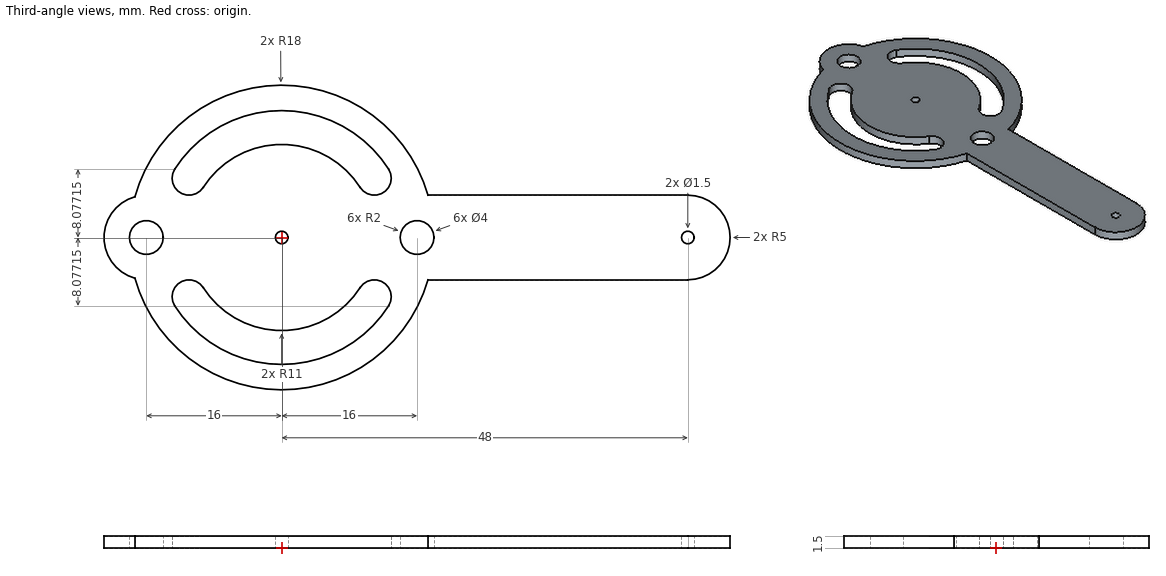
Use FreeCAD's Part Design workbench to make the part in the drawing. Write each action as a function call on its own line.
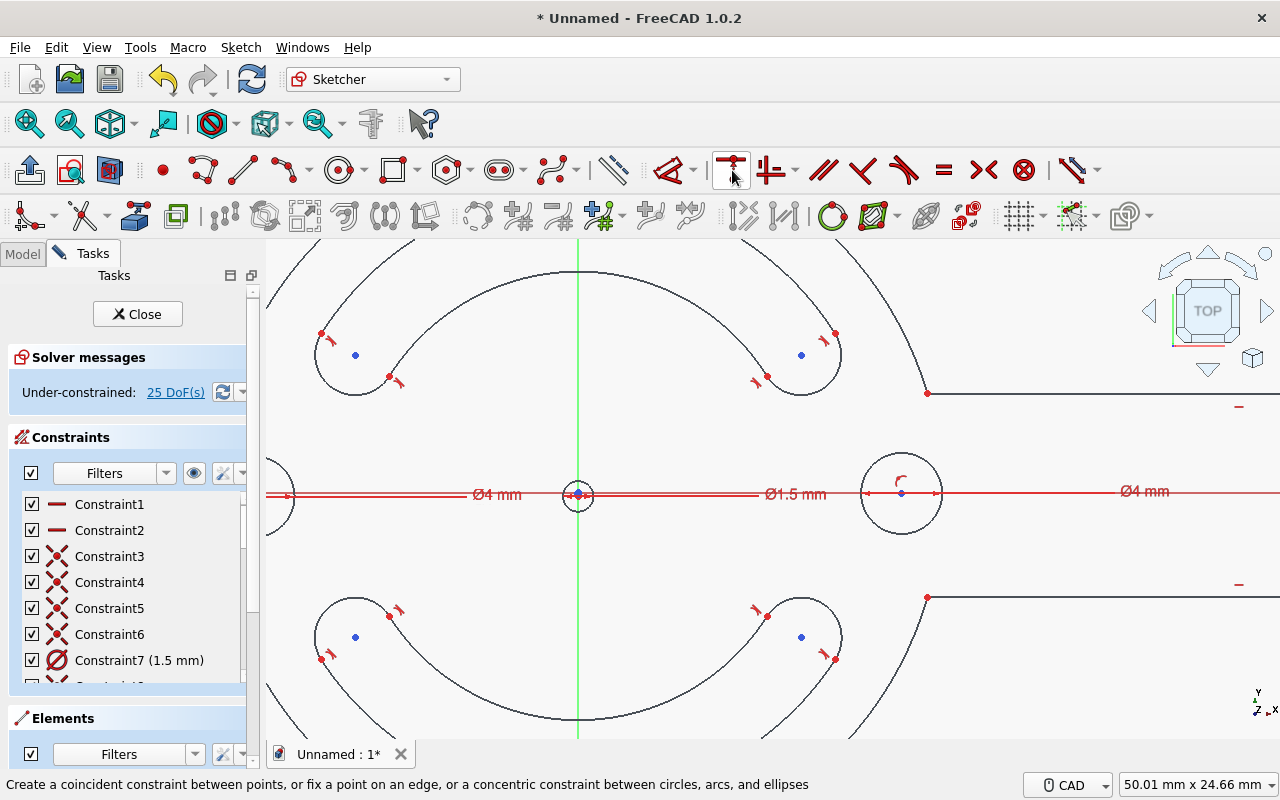
scroll(567, 507, up, 2)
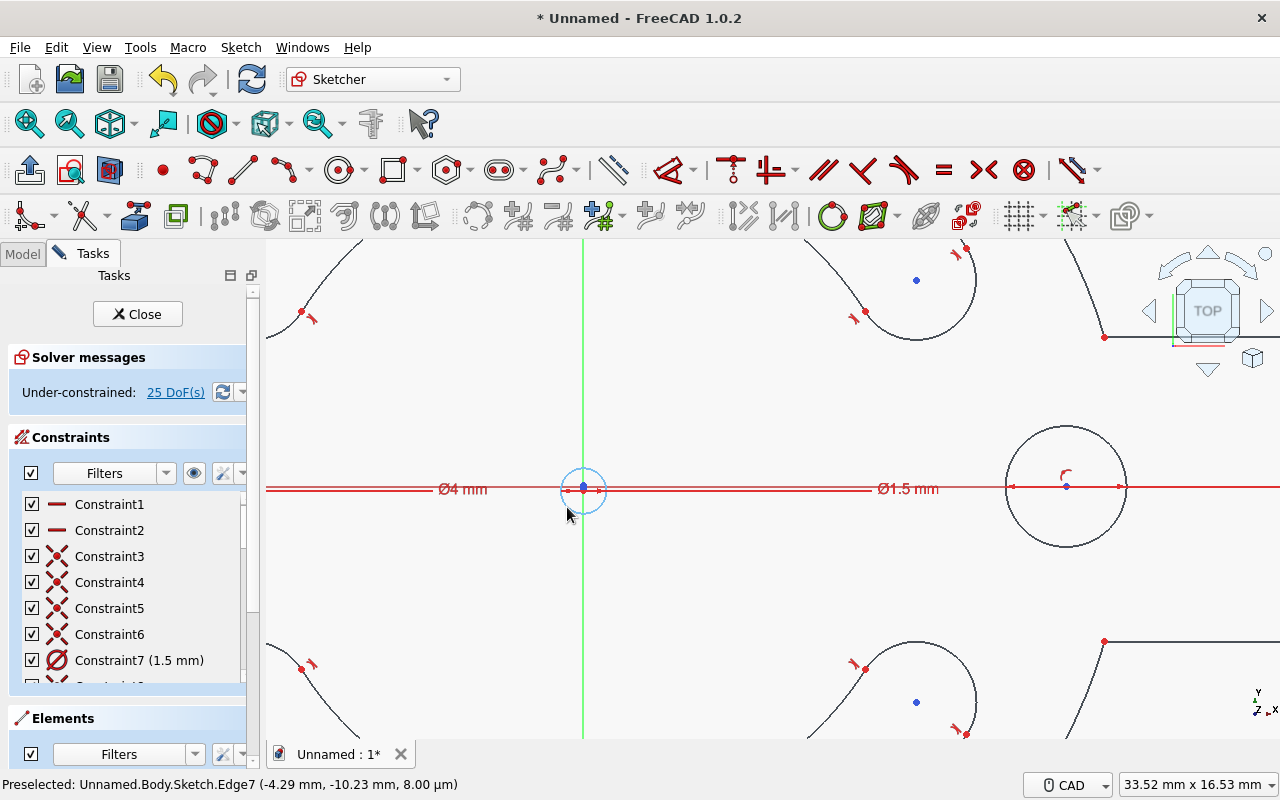
click(568, 507)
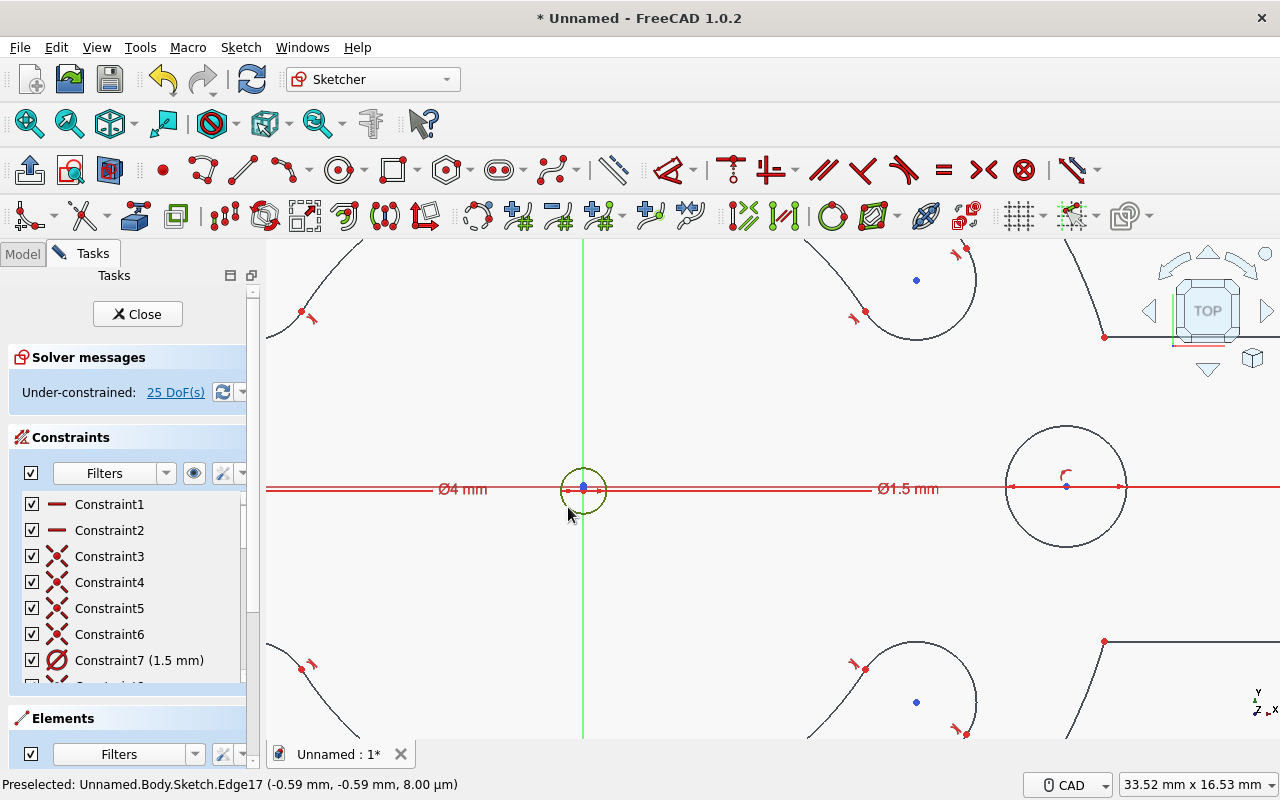
scroll(586, 490, down, 7)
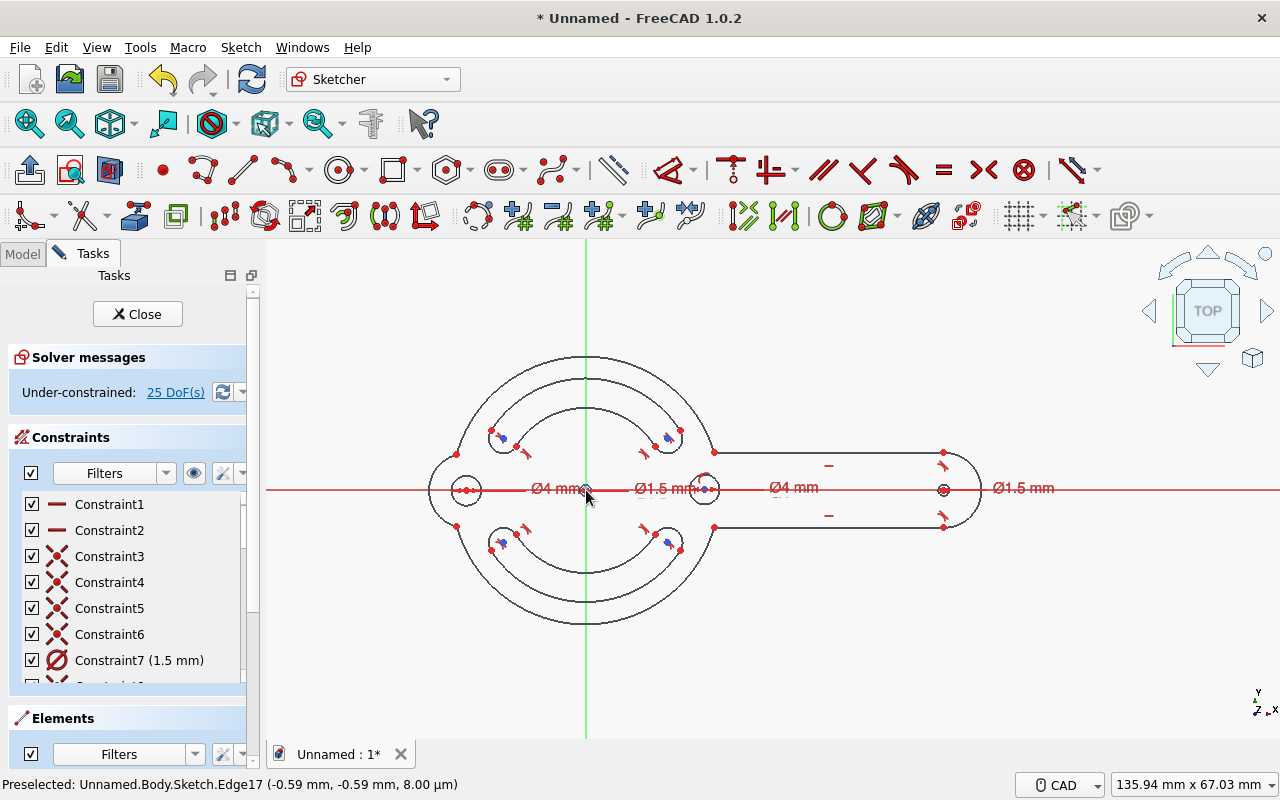
click(542, 593)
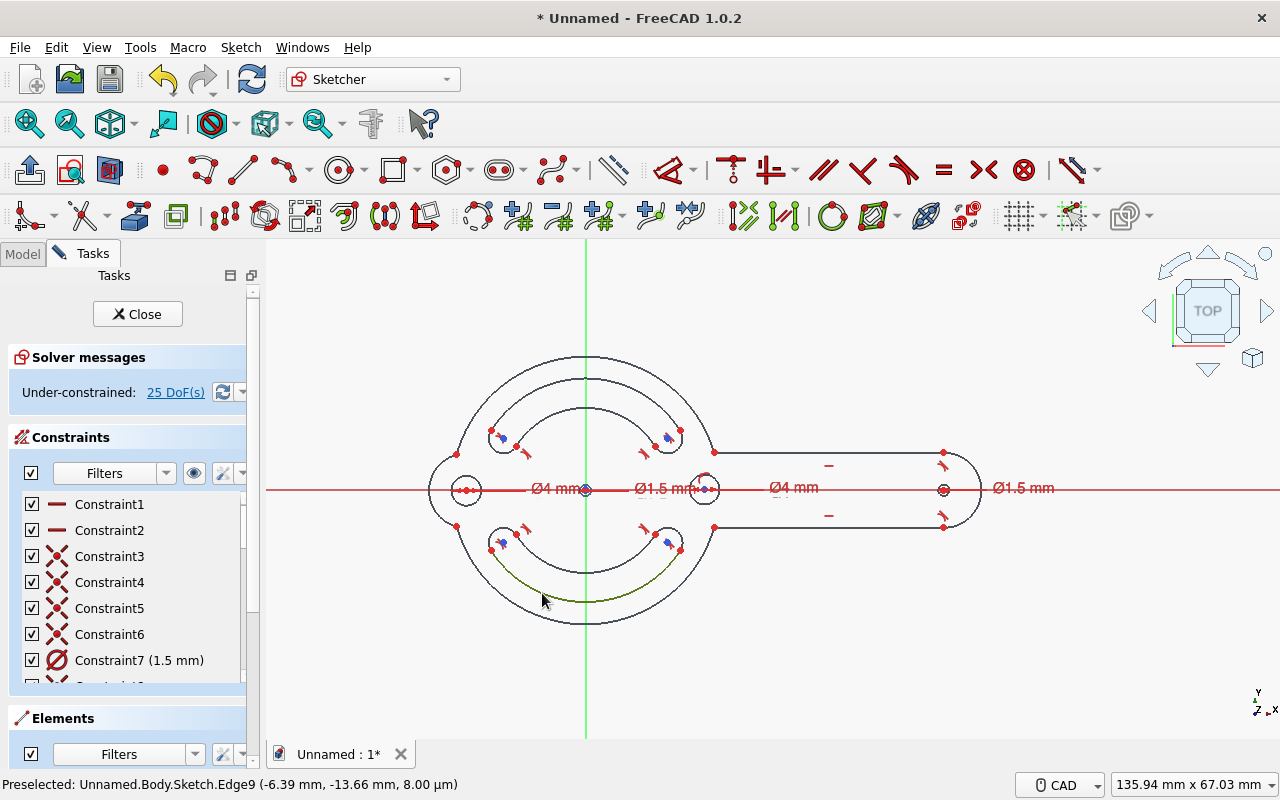
click(732, 170)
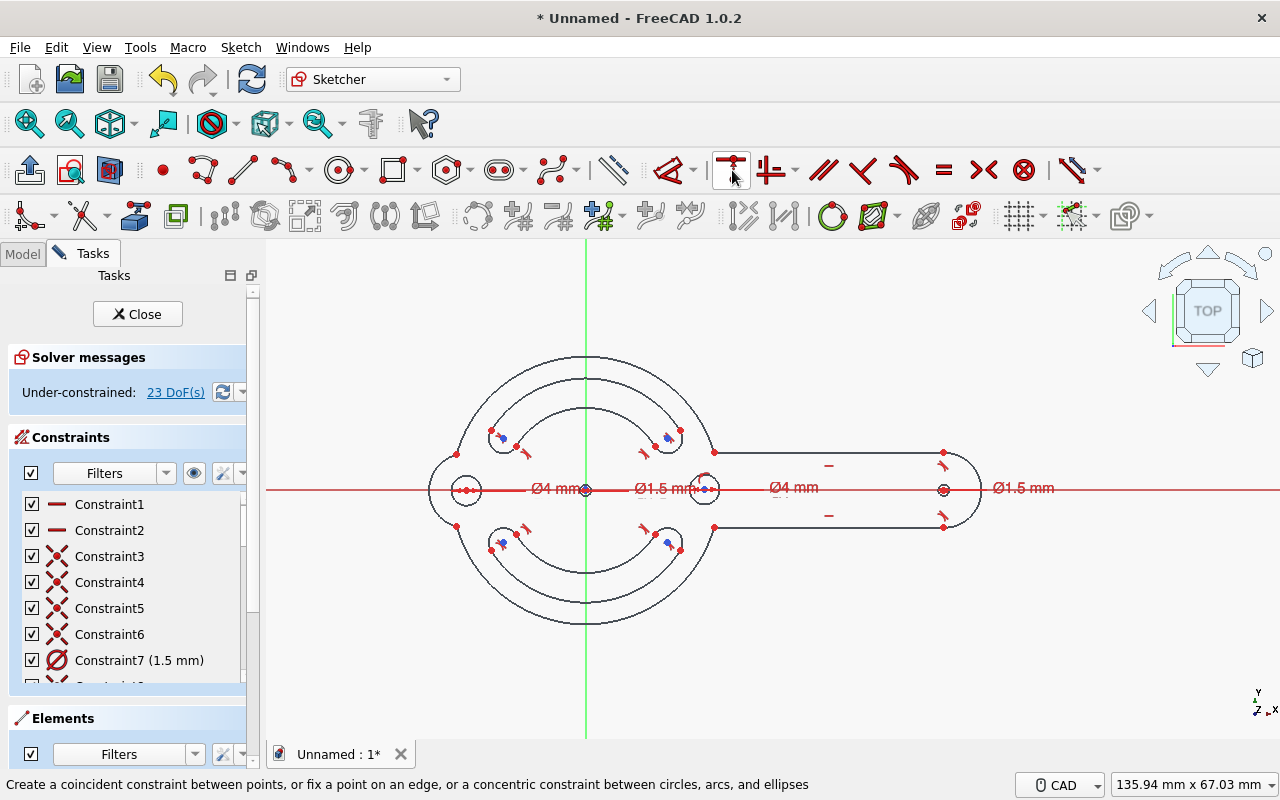
scroll(582, 487, up, 5)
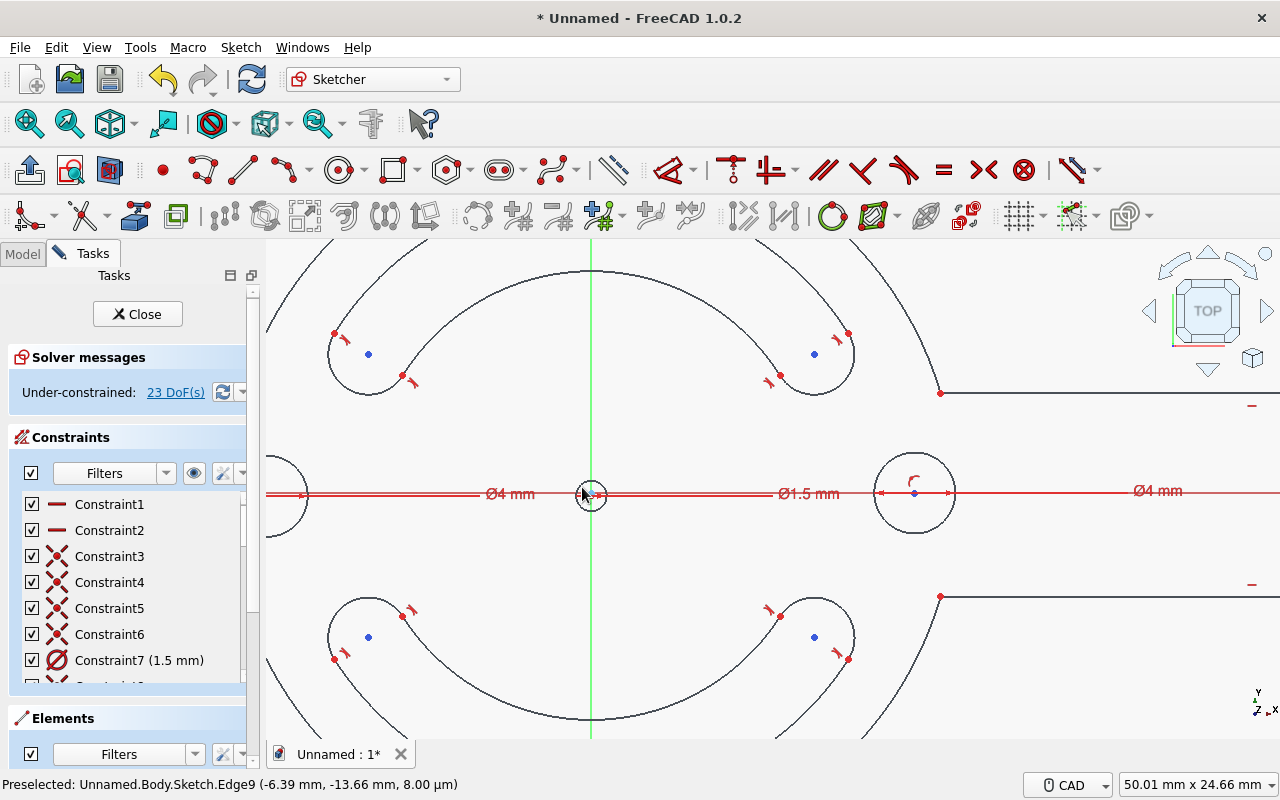
click(581, 485)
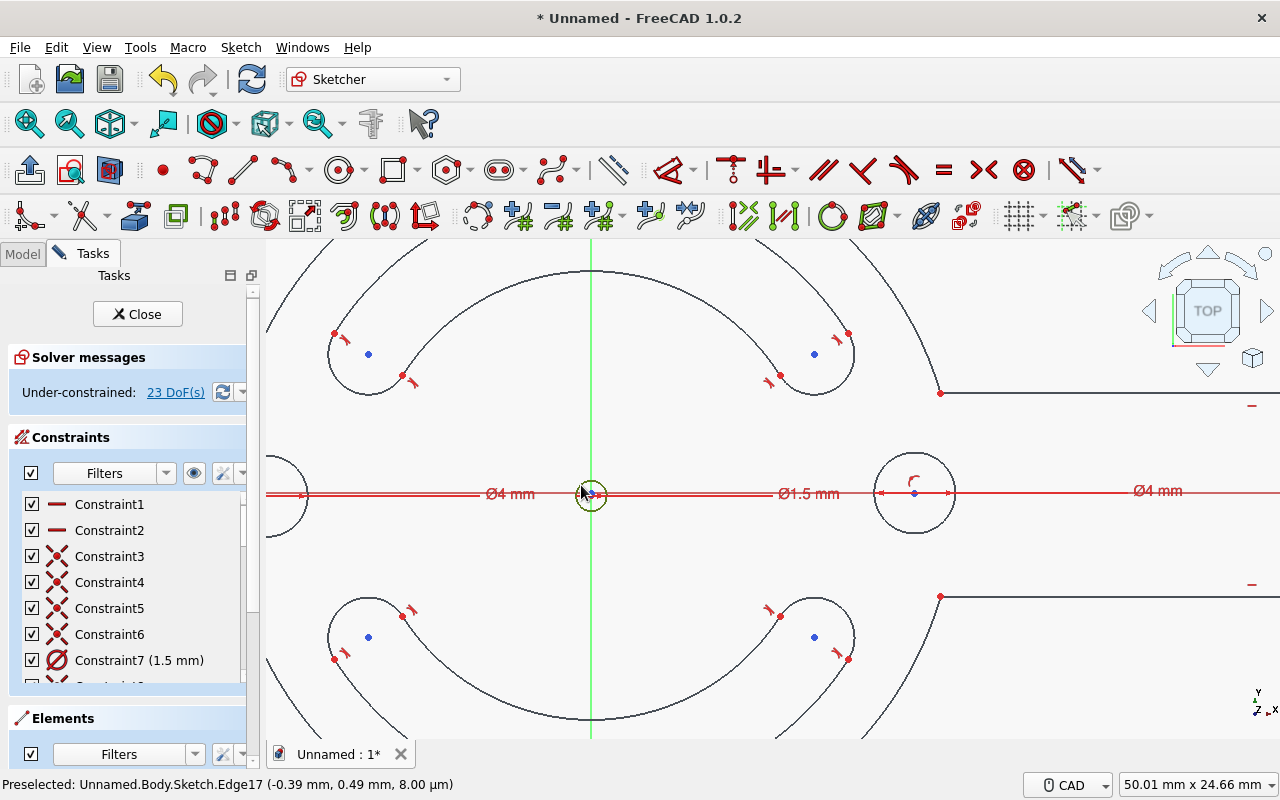
click(679, 289)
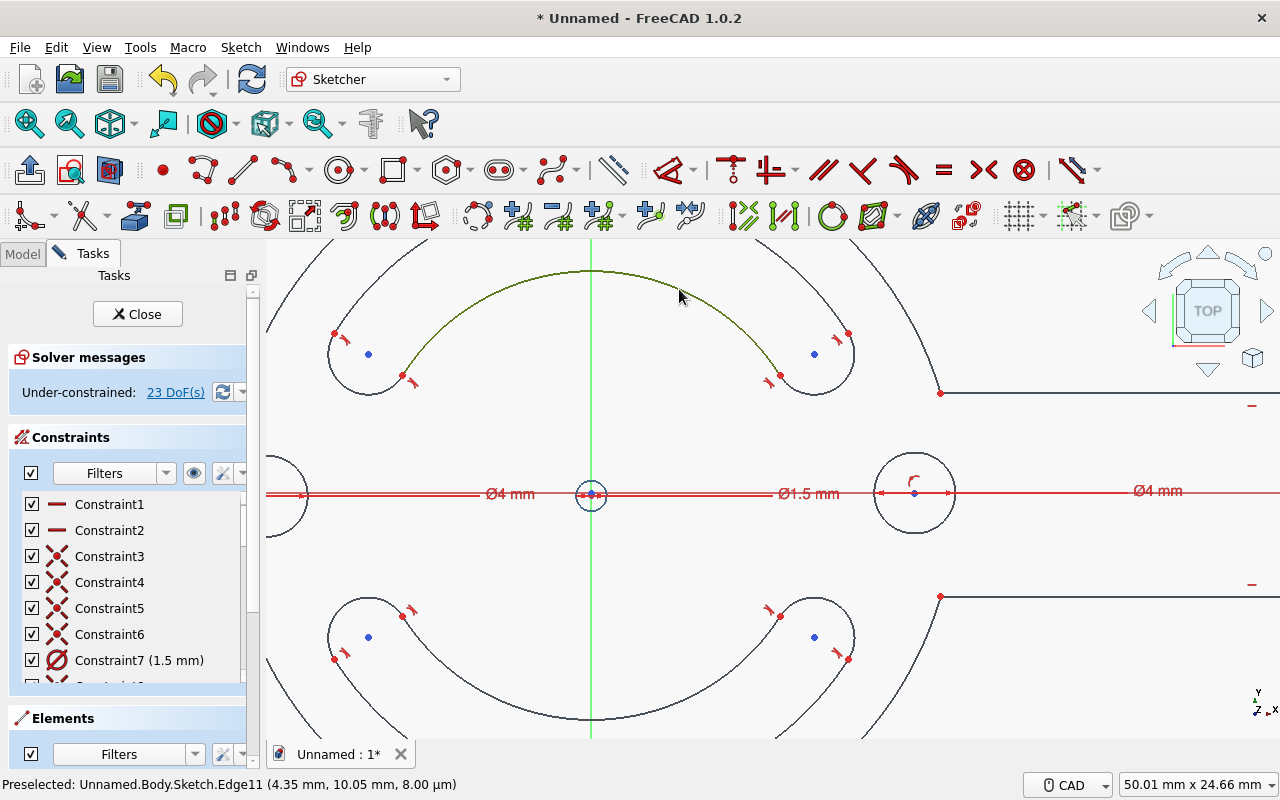
click(732, 170)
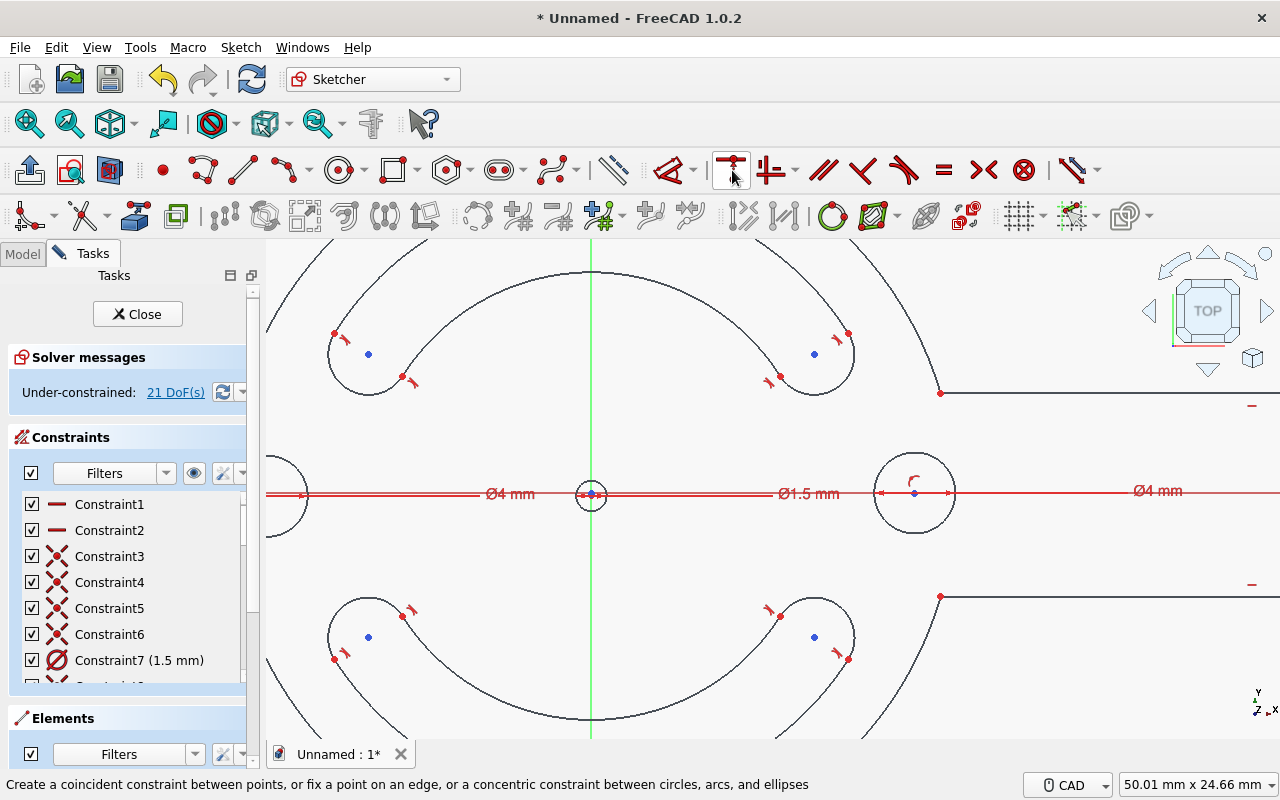
scroll(581, 507, up, 2)